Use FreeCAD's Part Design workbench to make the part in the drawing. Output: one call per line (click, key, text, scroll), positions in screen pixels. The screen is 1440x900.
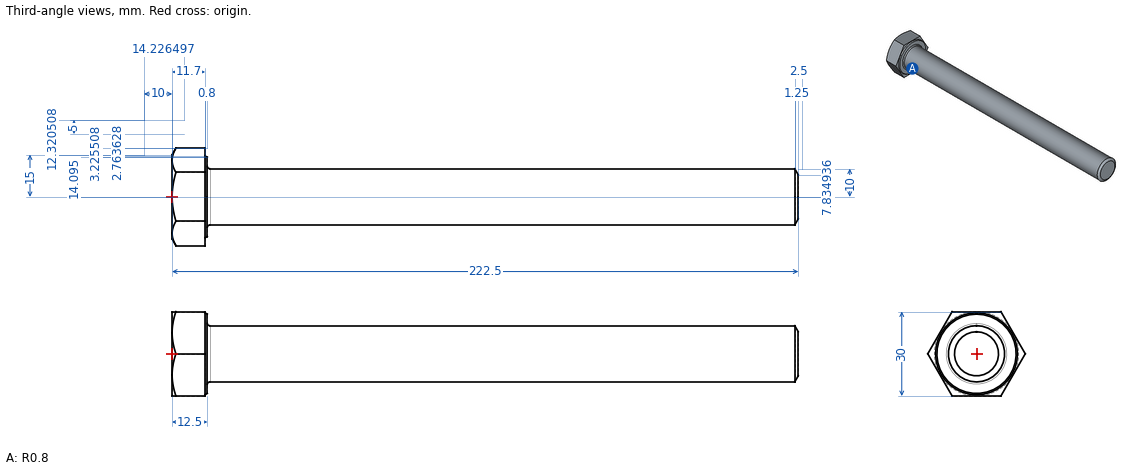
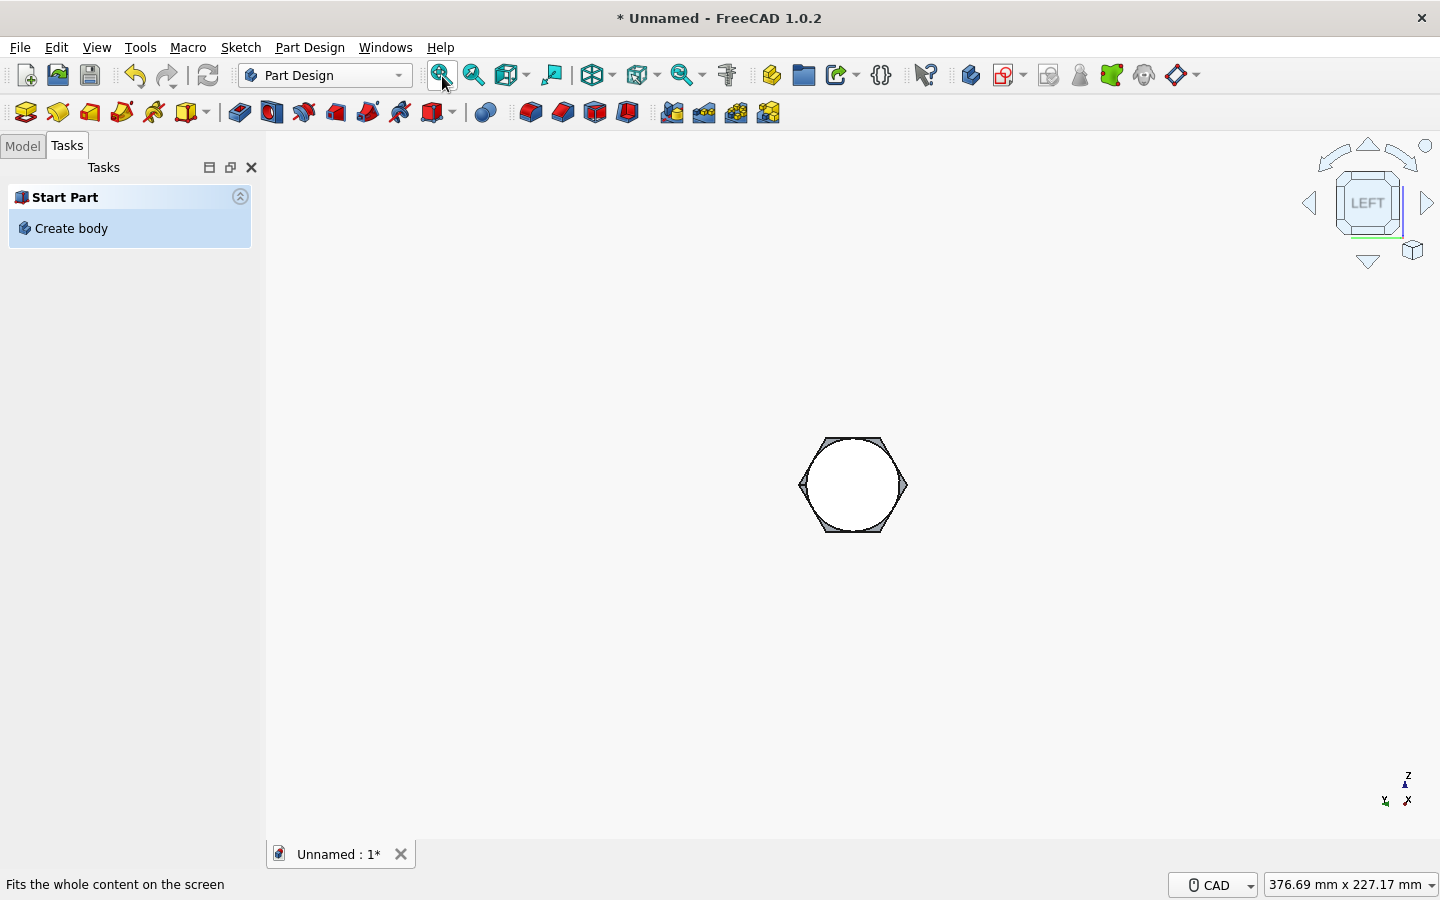
key(0)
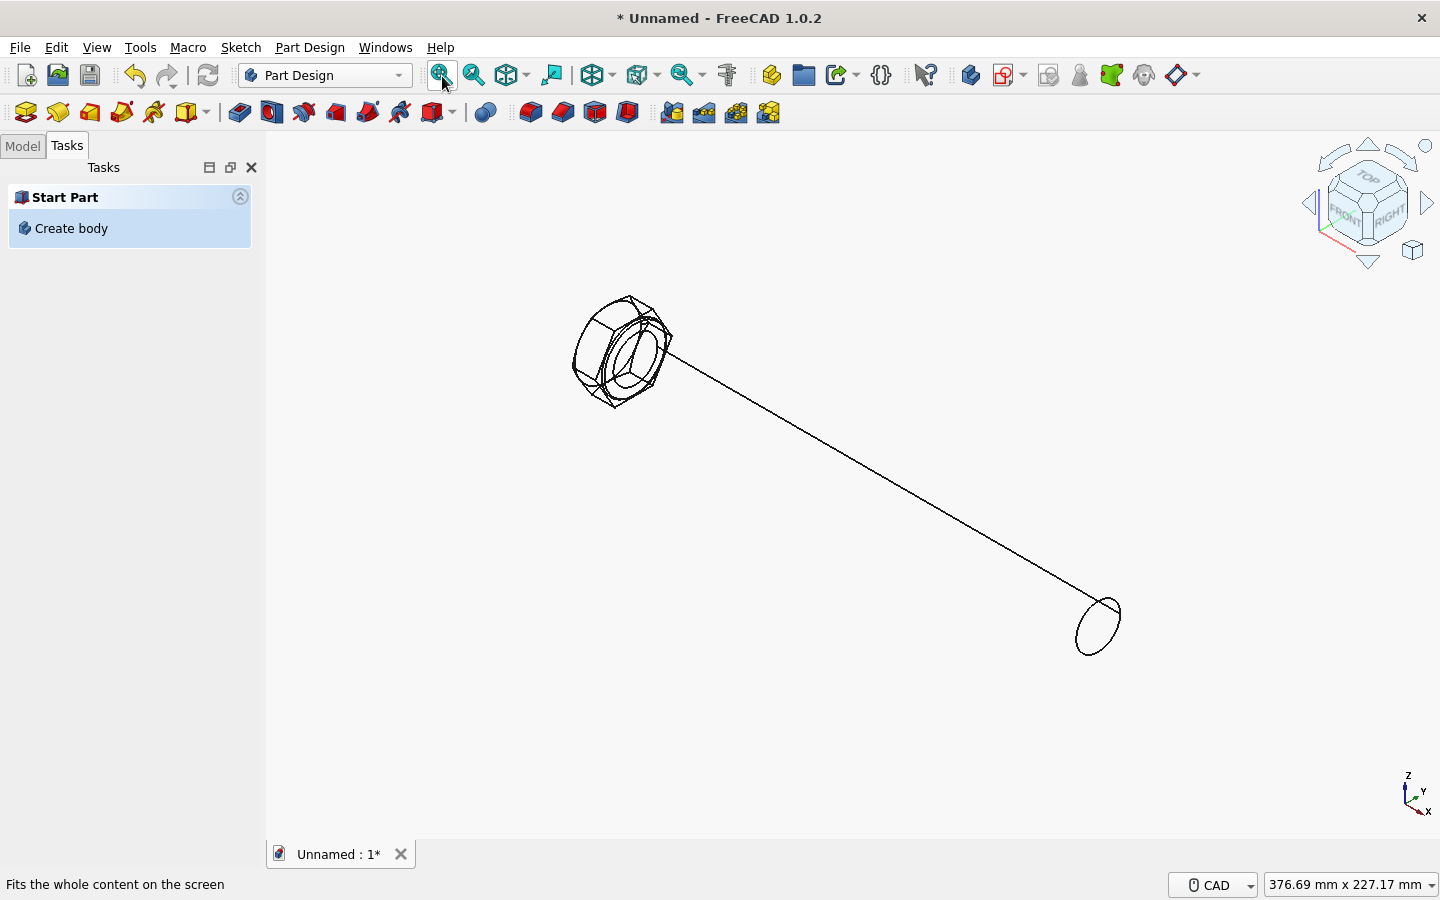
click(613, 371)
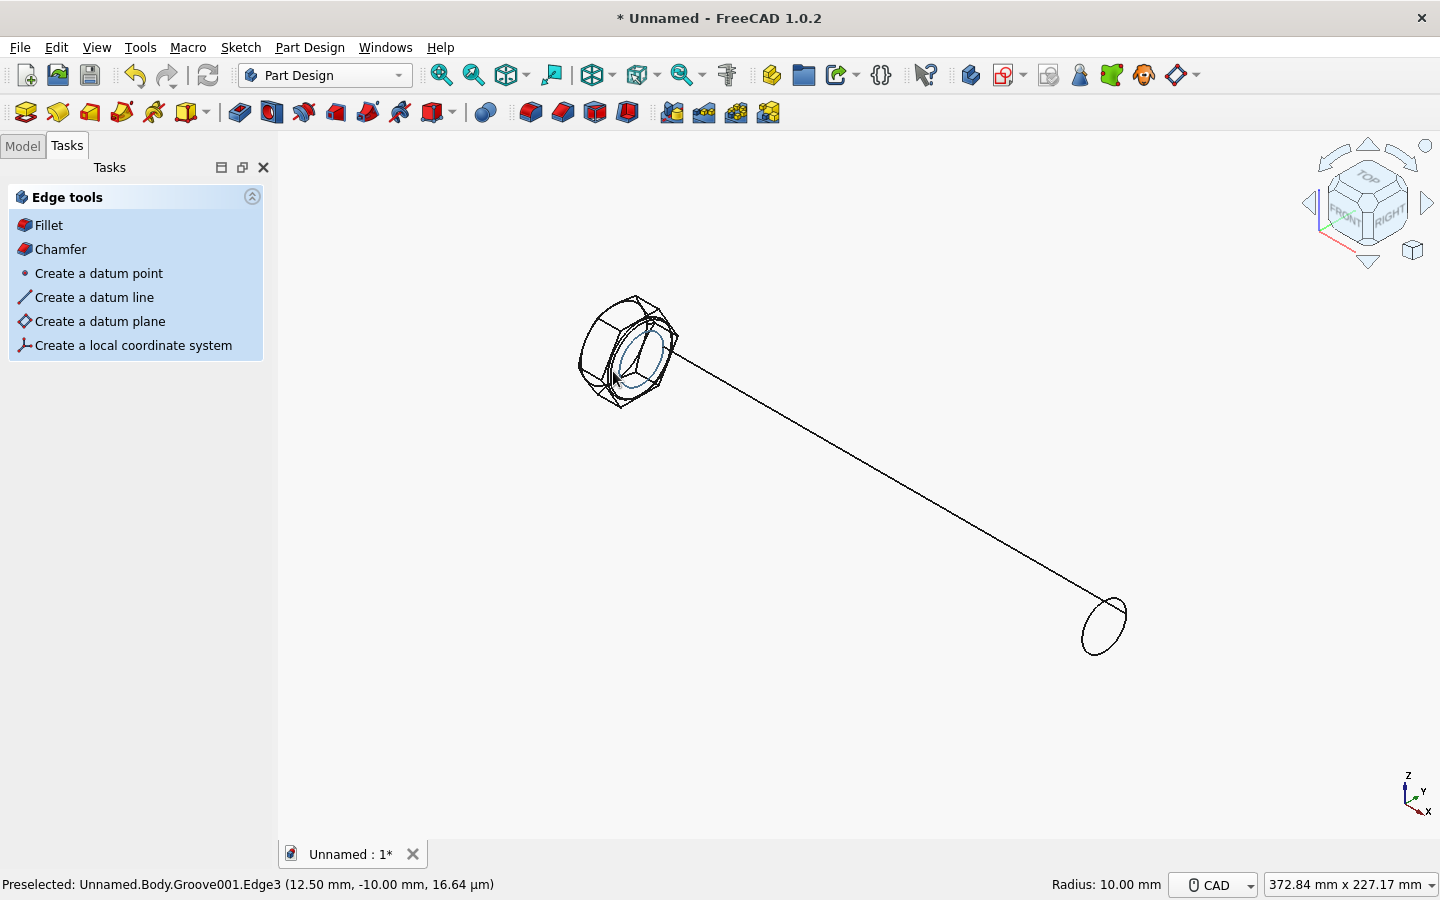
key(v)
key(1)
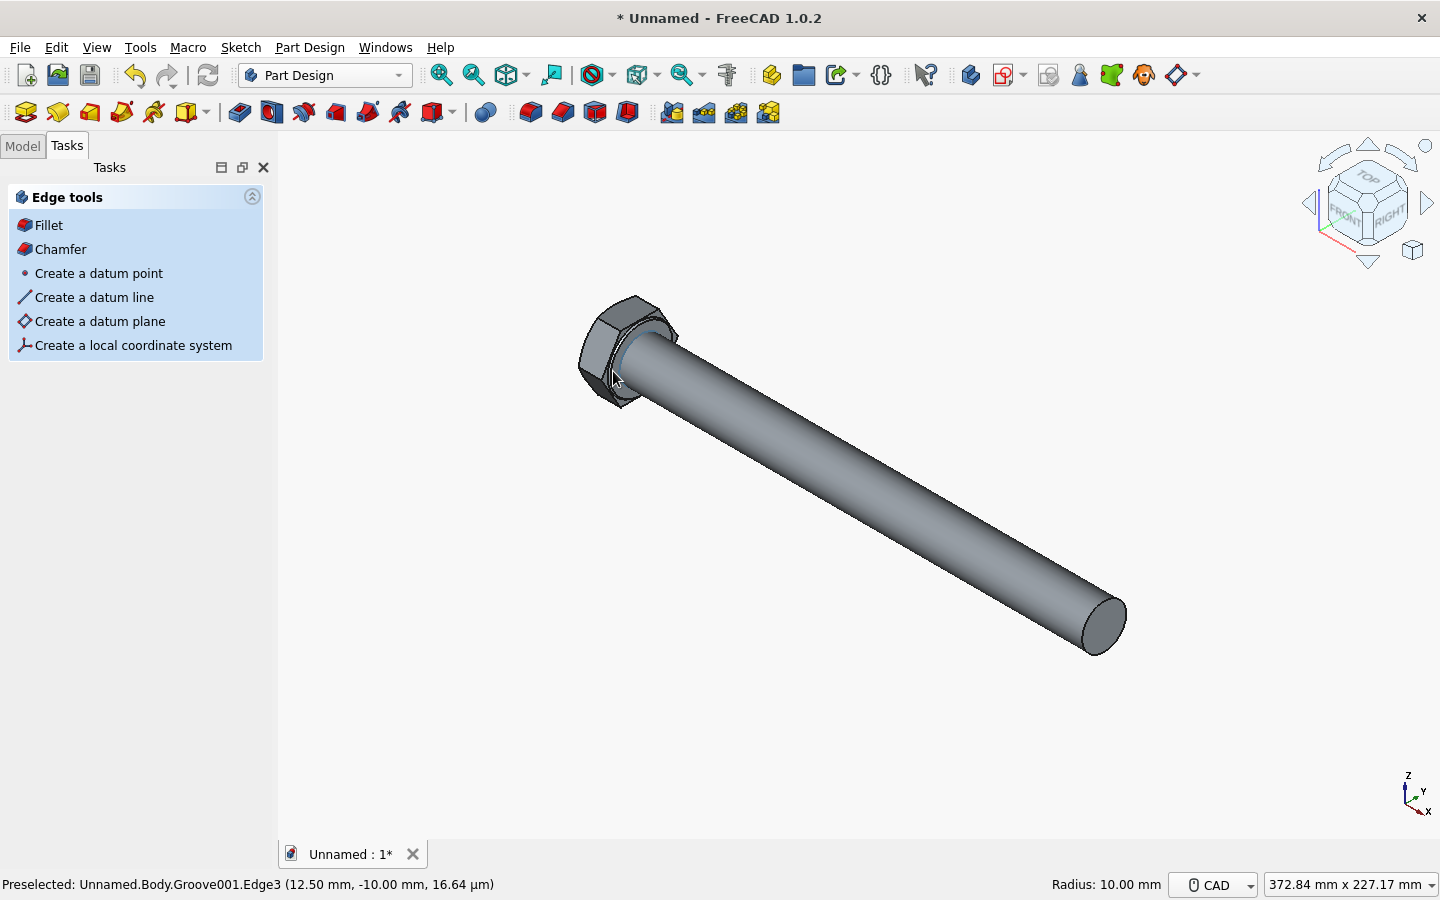
click(532, 112)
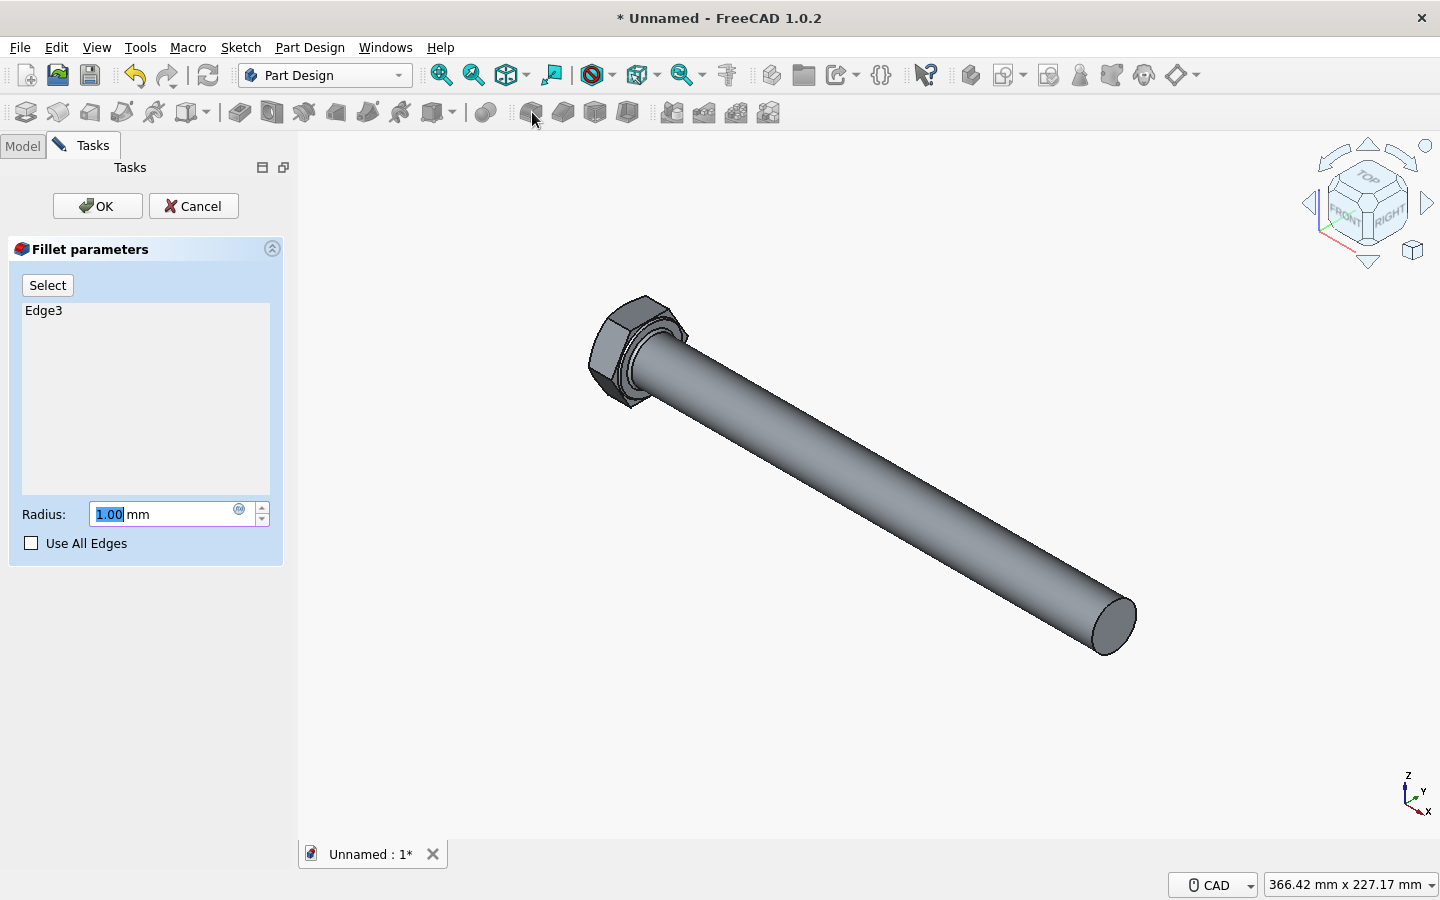
text(0.8)
key(Tab)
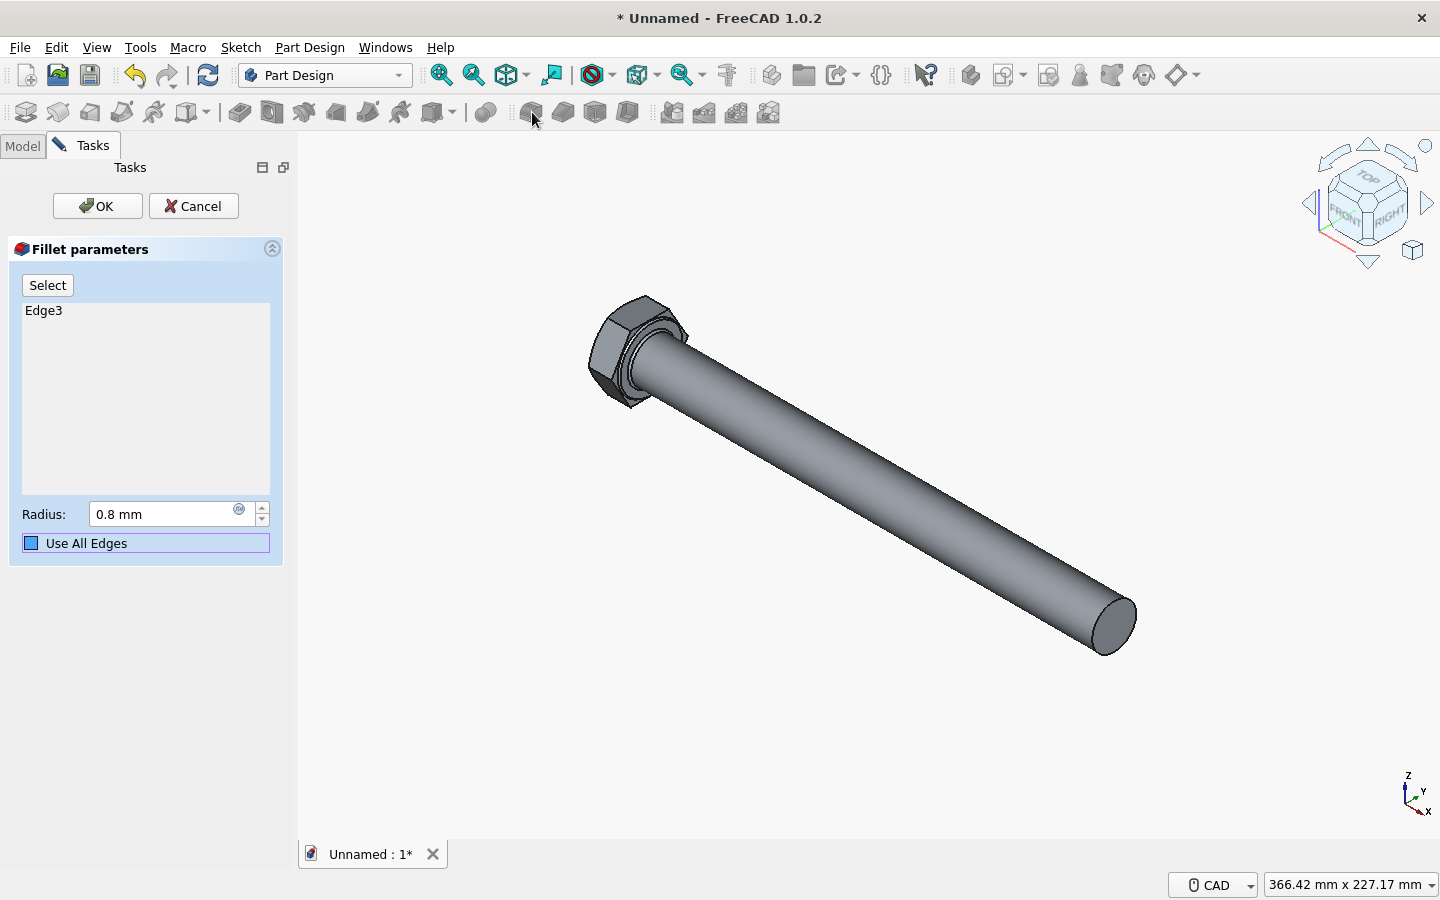
click(98, 206)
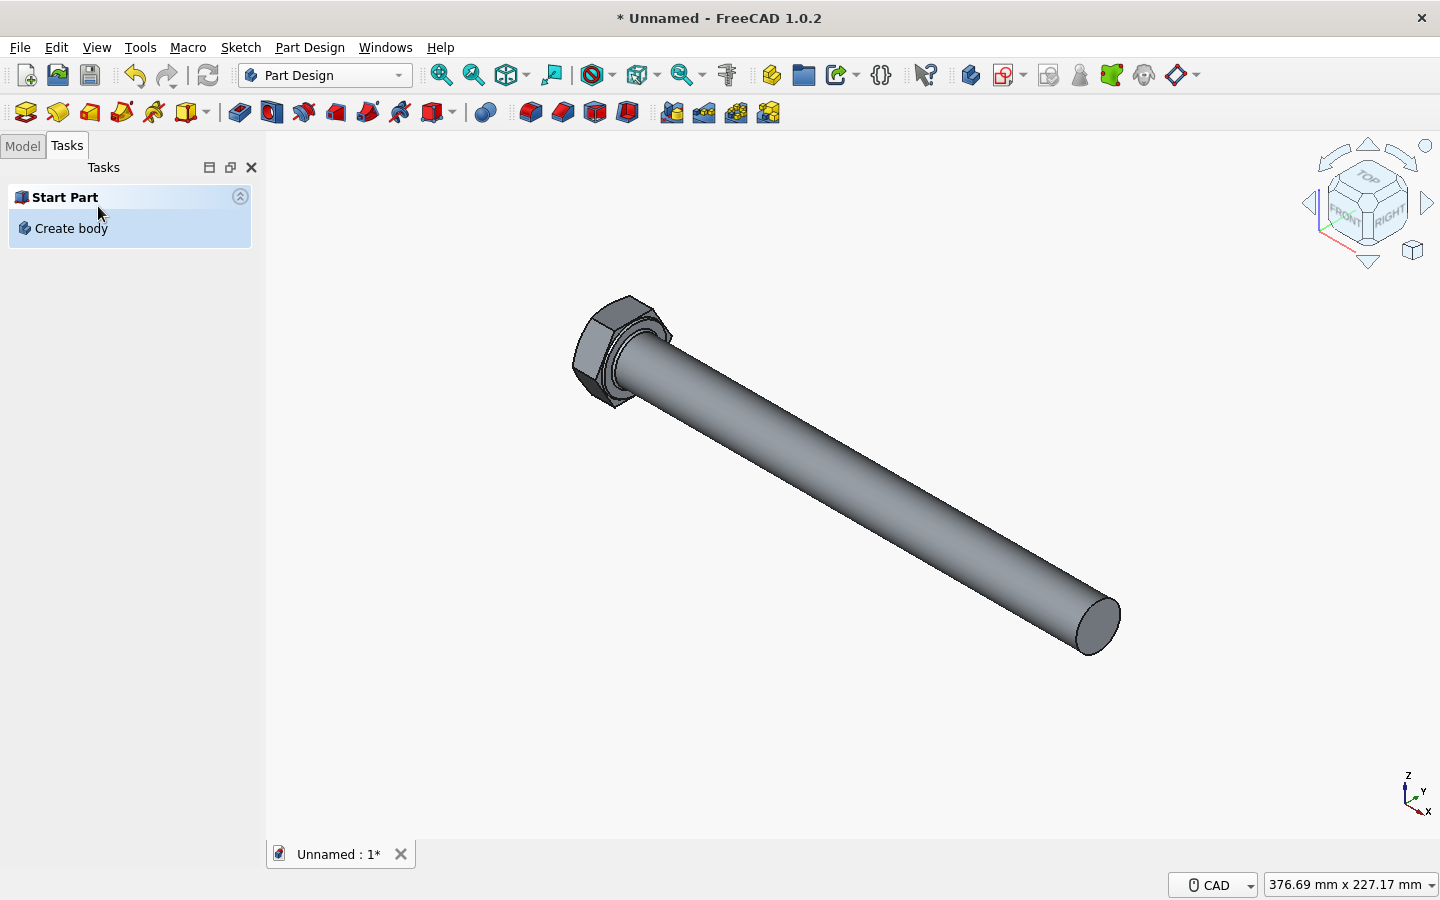
click(1004, 76)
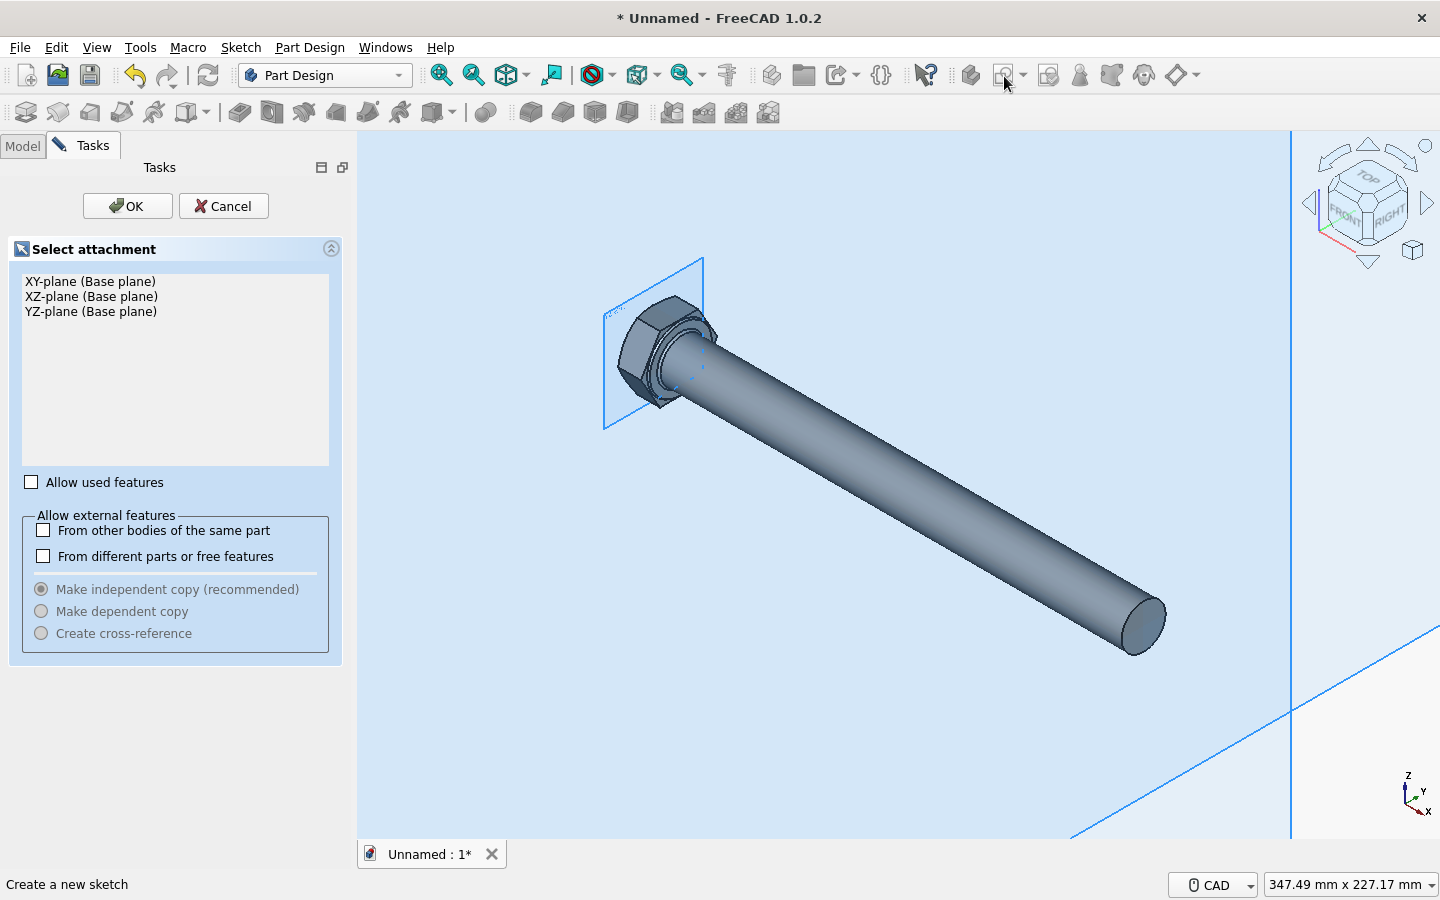
click(82, 282)